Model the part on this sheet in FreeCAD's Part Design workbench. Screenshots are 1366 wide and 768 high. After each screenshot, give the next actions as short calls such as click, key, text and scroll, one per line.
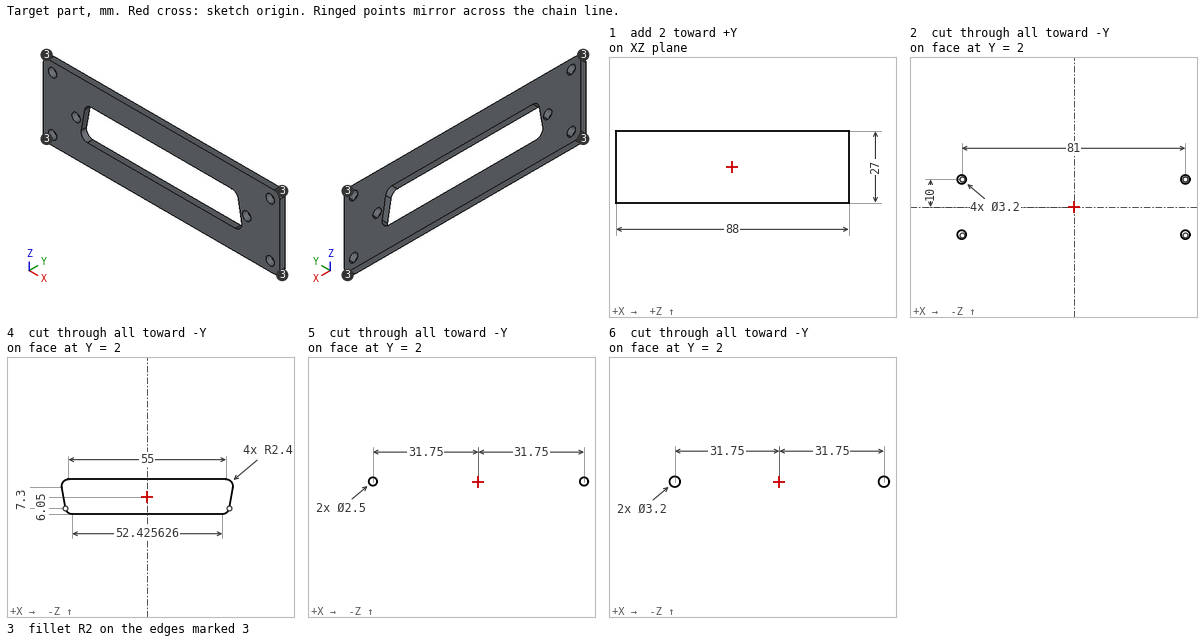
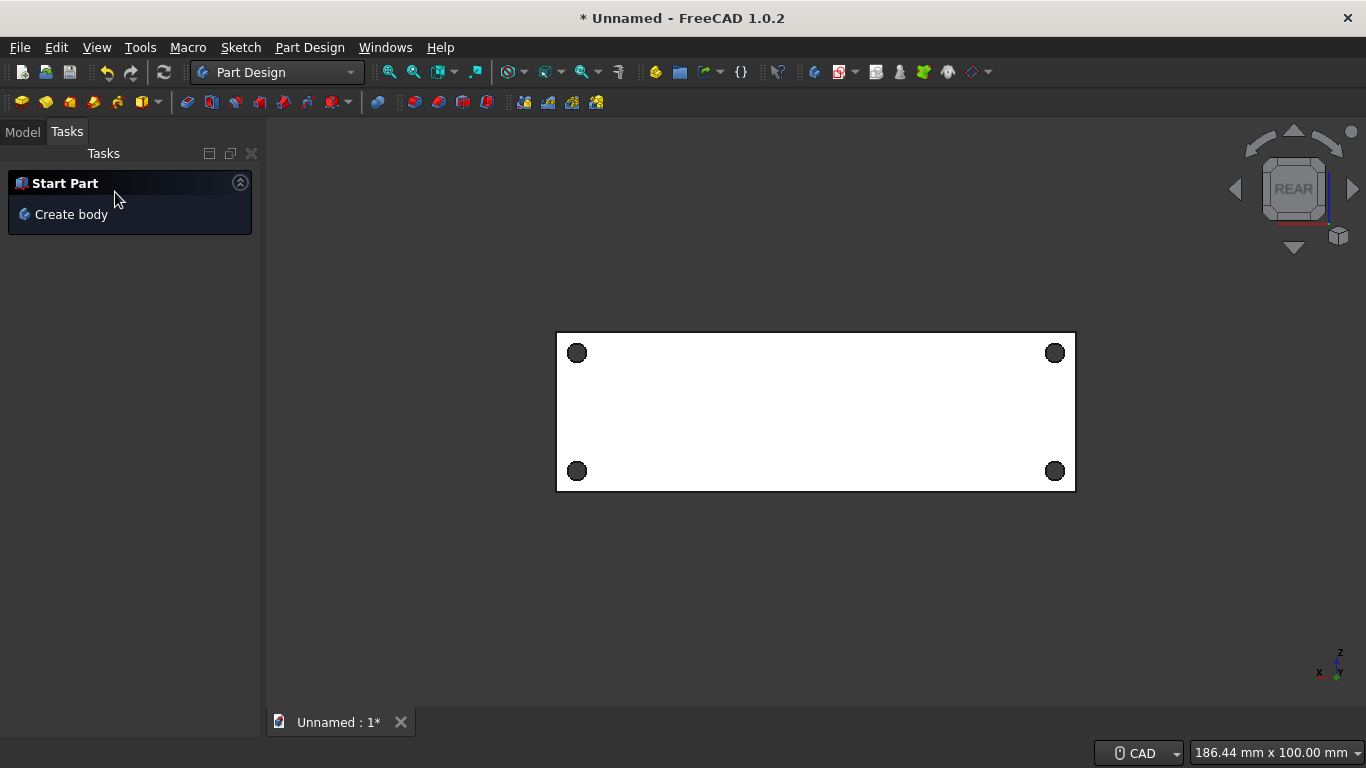
scroll(556, 331, up, 7)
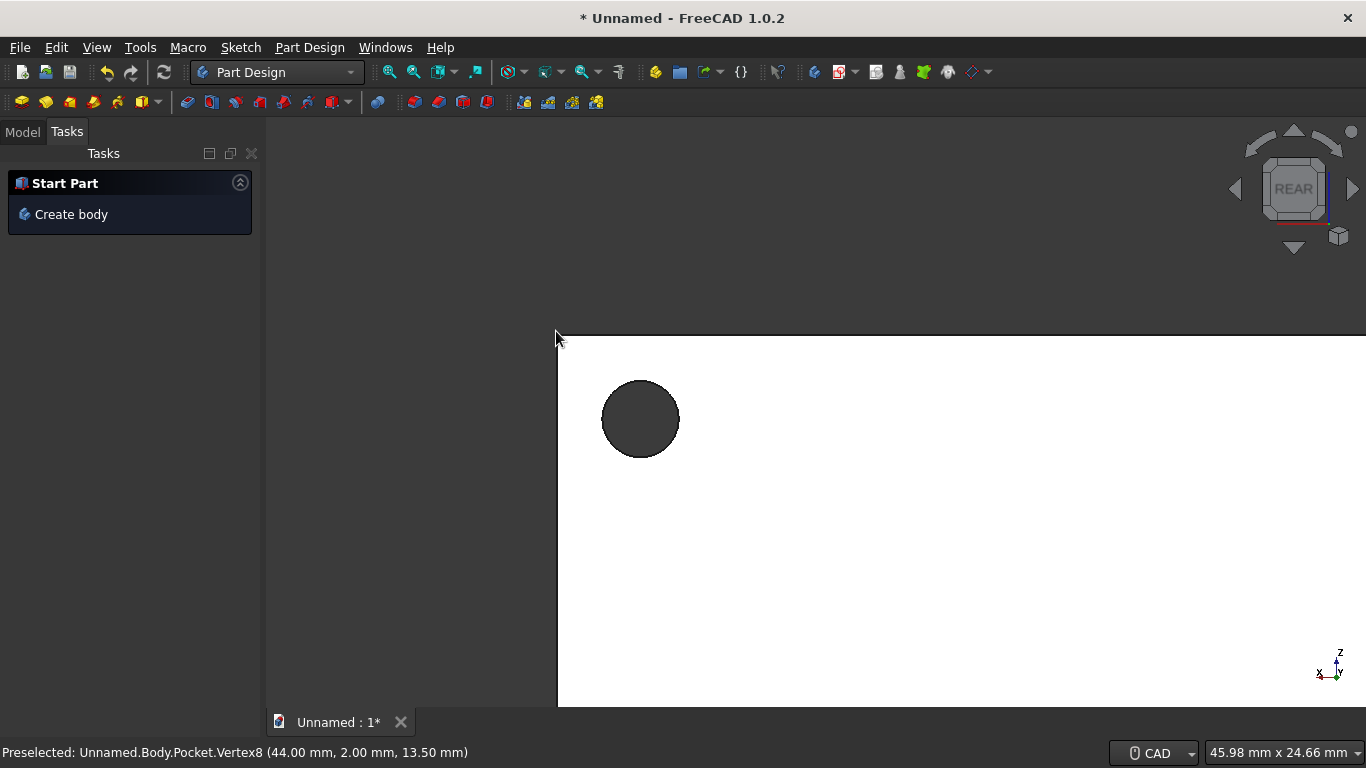
click(390, 72)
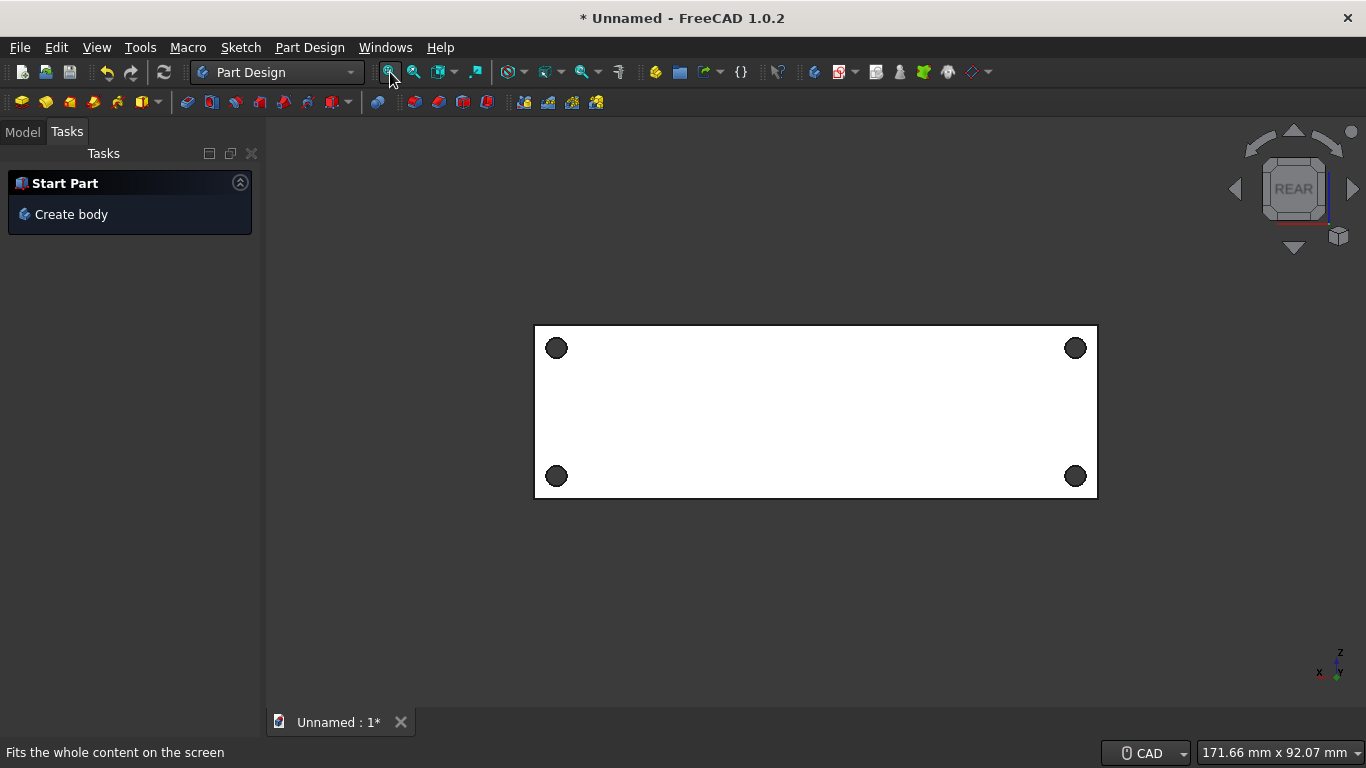
key(0)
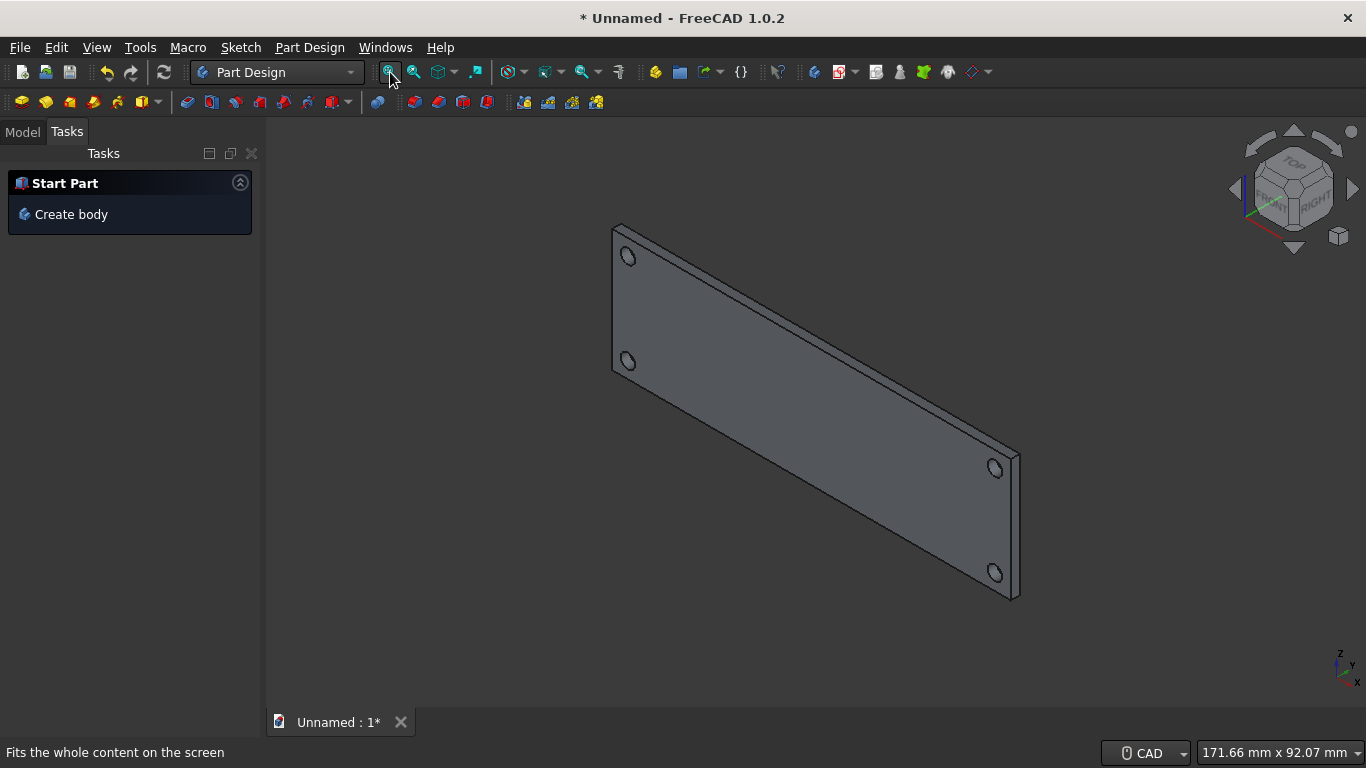
click(1017, 454)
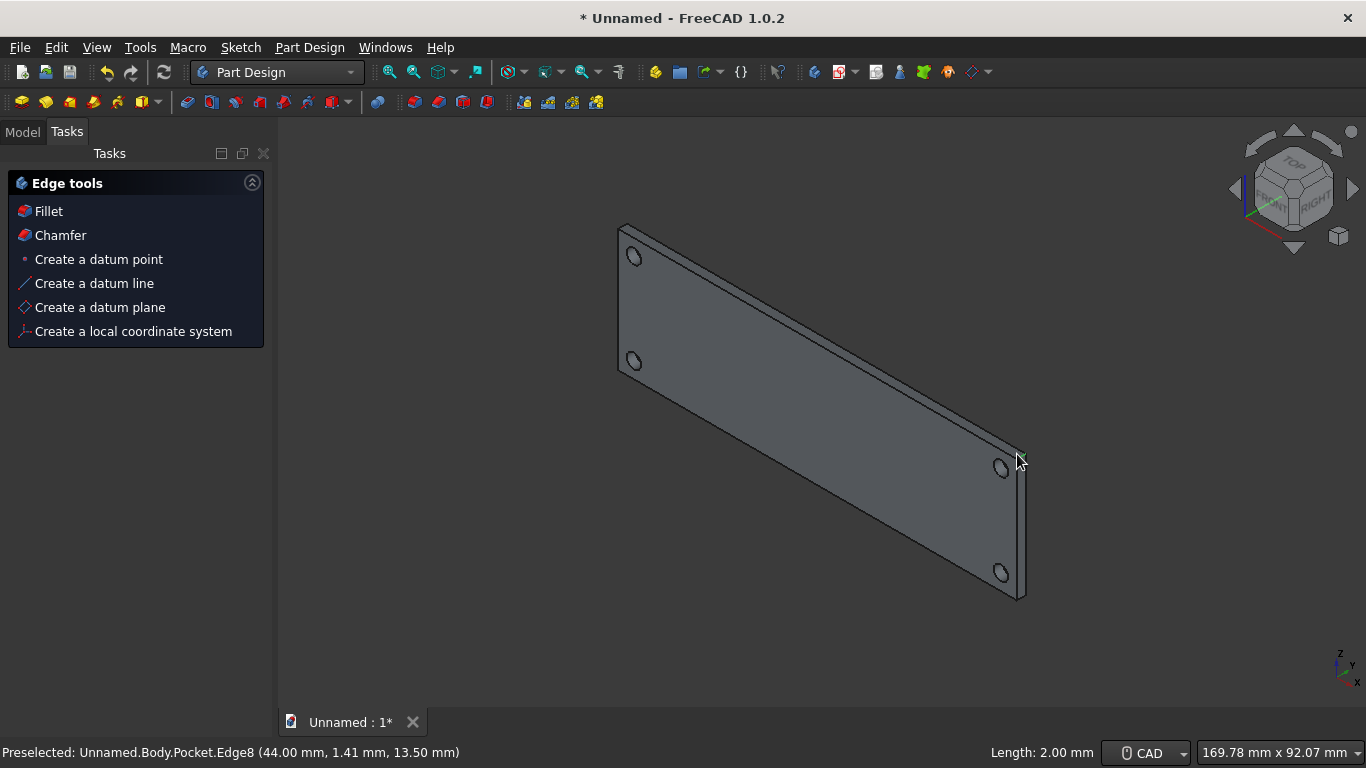
scroll(623, 225, up, 6)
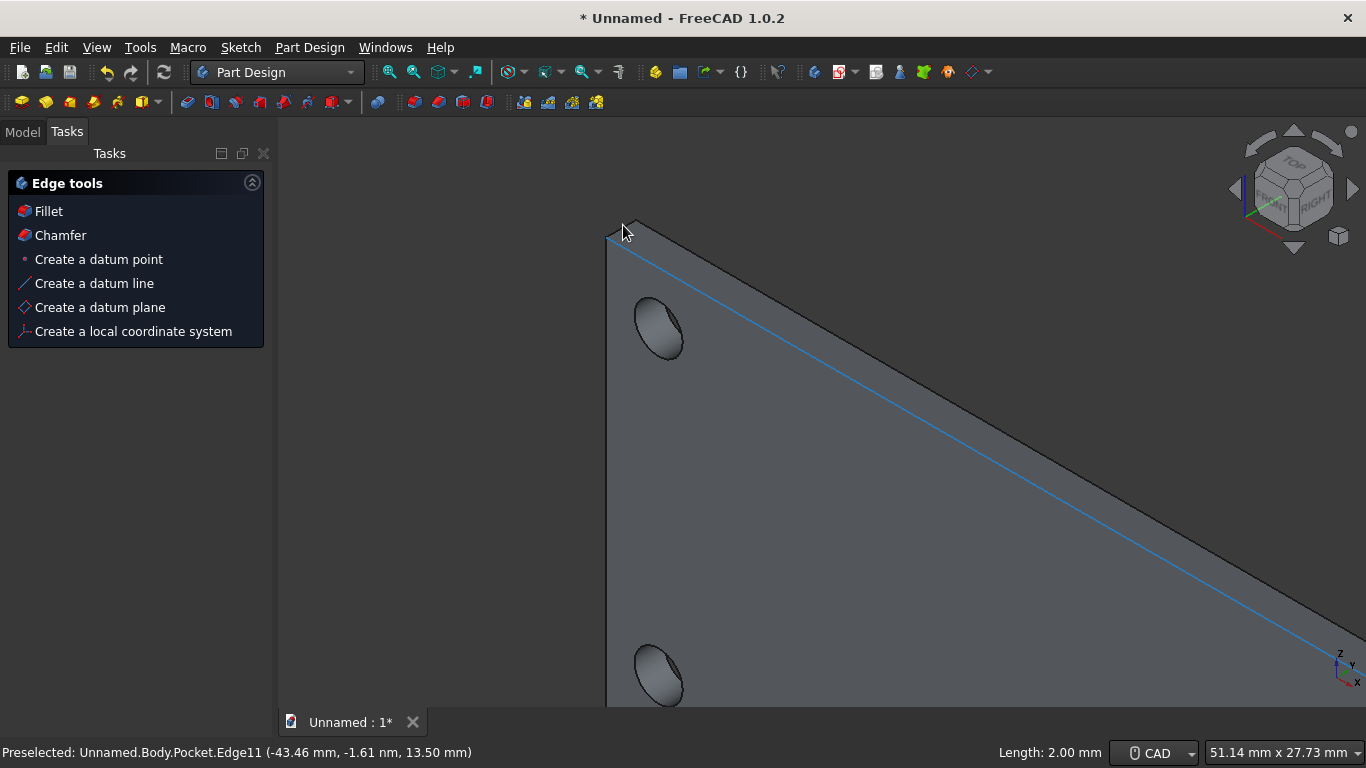
click(390, 72)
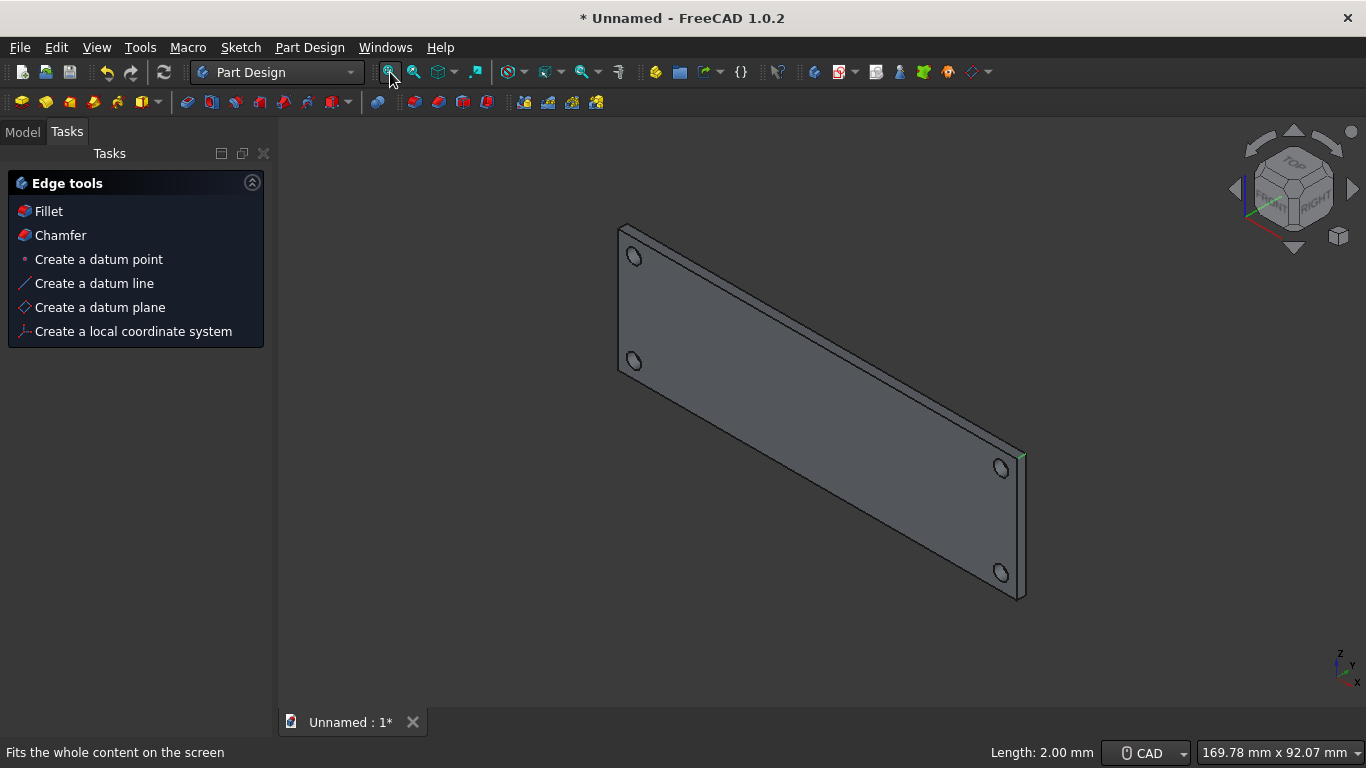
key(2)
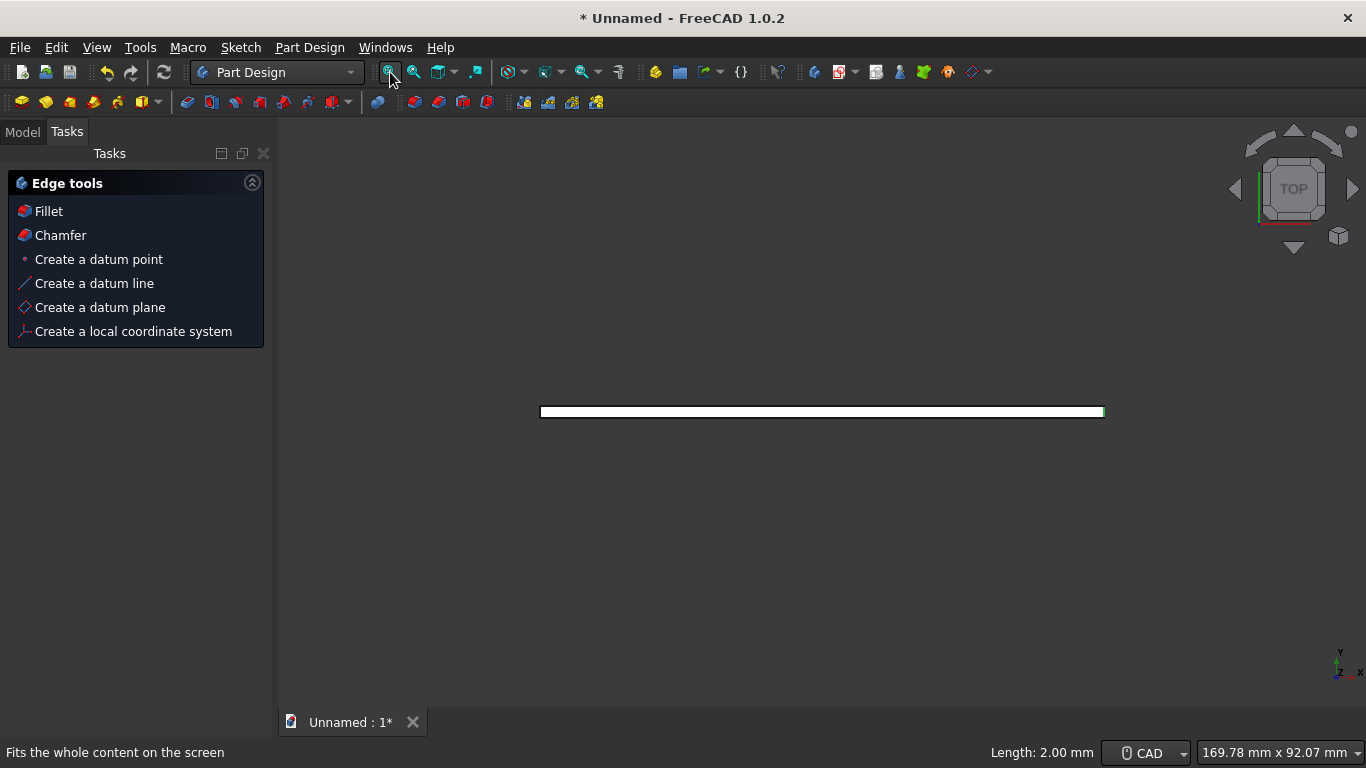
click(540, 411, ctrl)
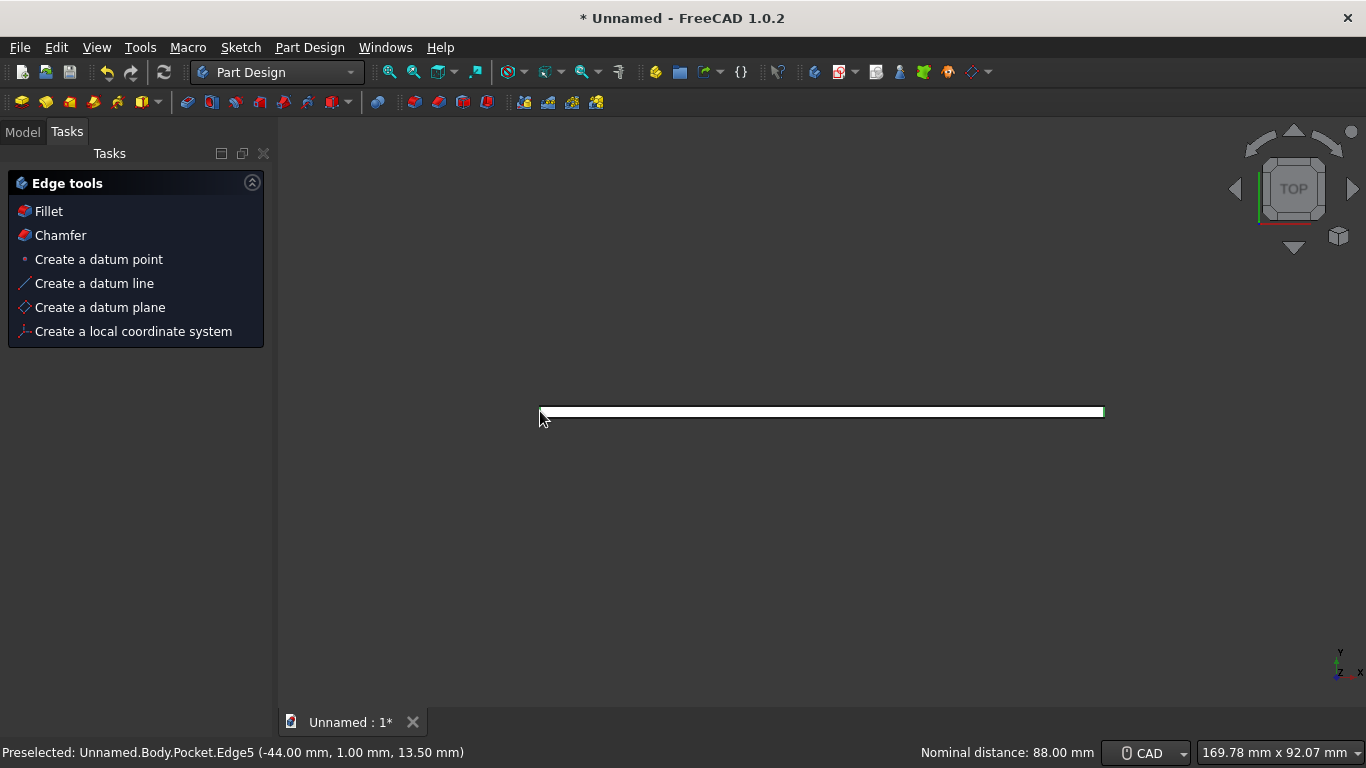
scroll(540, 411, up, 6)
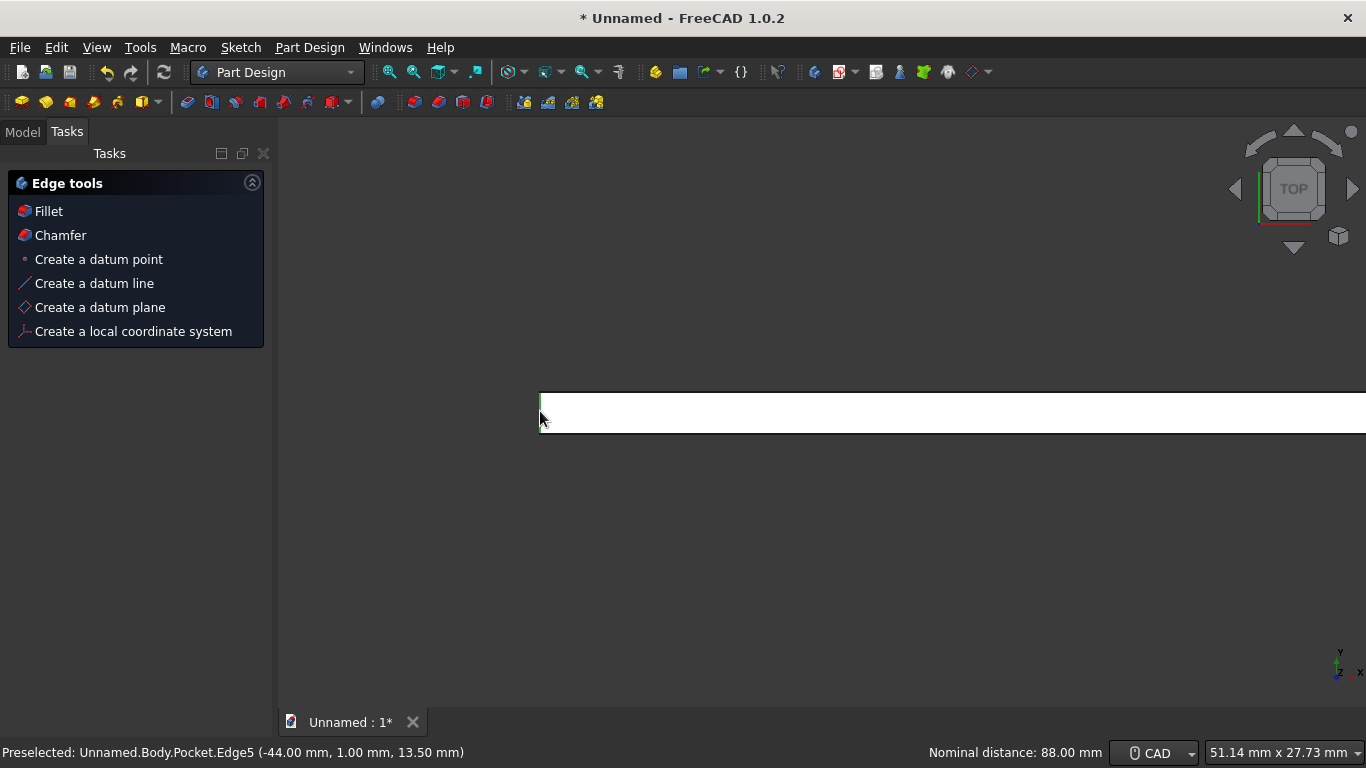
click(390, 72)